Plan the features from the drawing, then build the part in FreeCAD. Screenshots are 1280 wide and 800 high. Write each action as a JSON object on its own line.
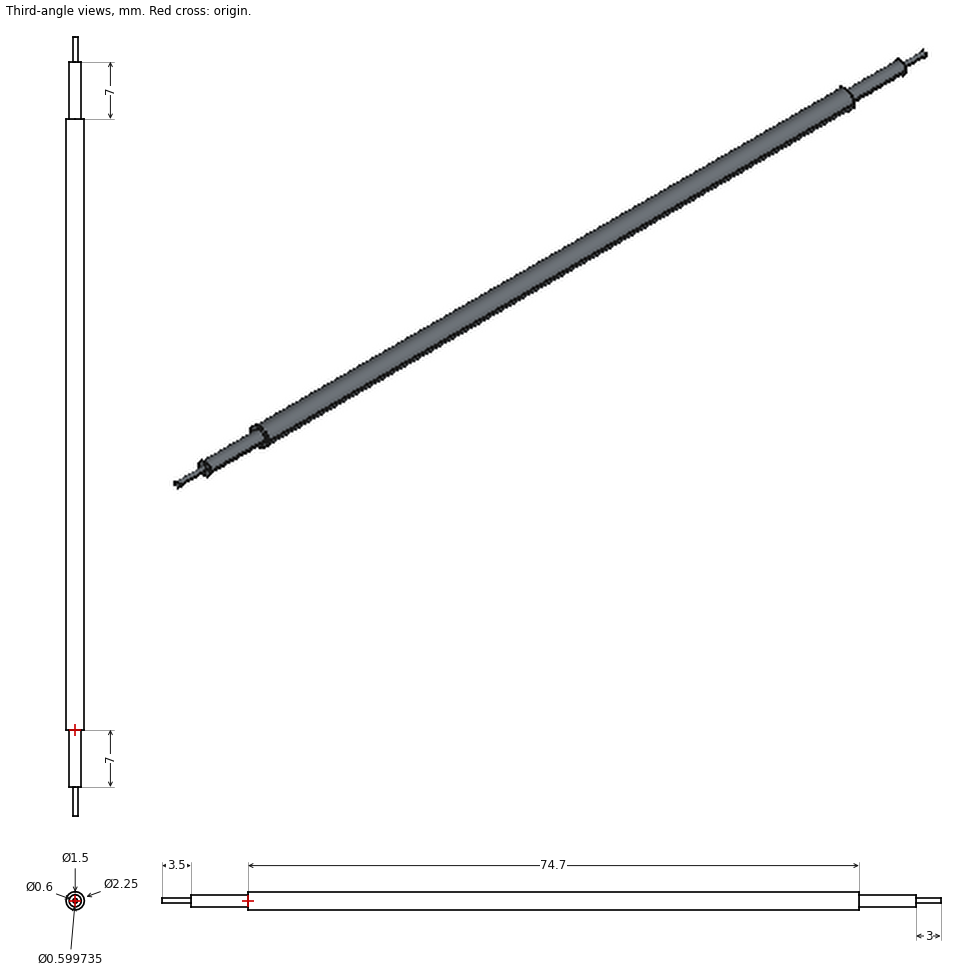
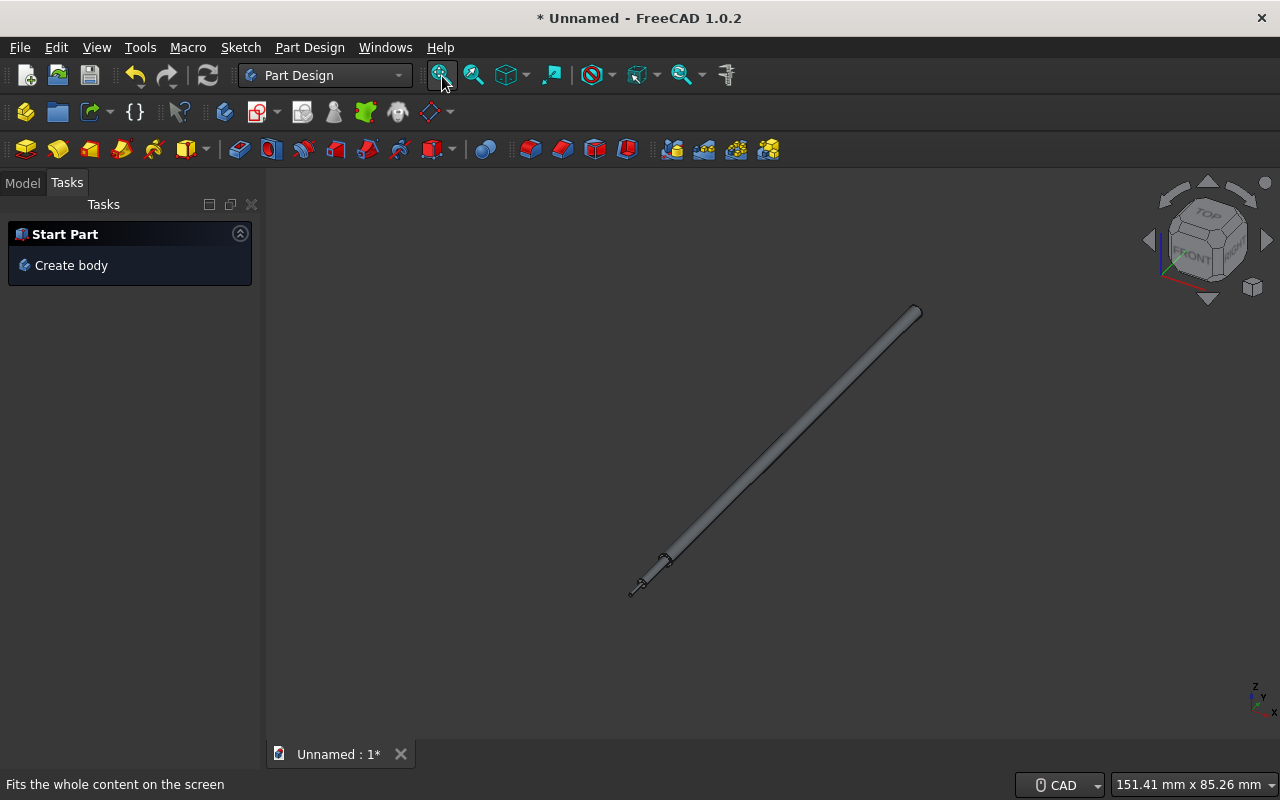
{"action": "left_click", "coordinate": [23, 182]}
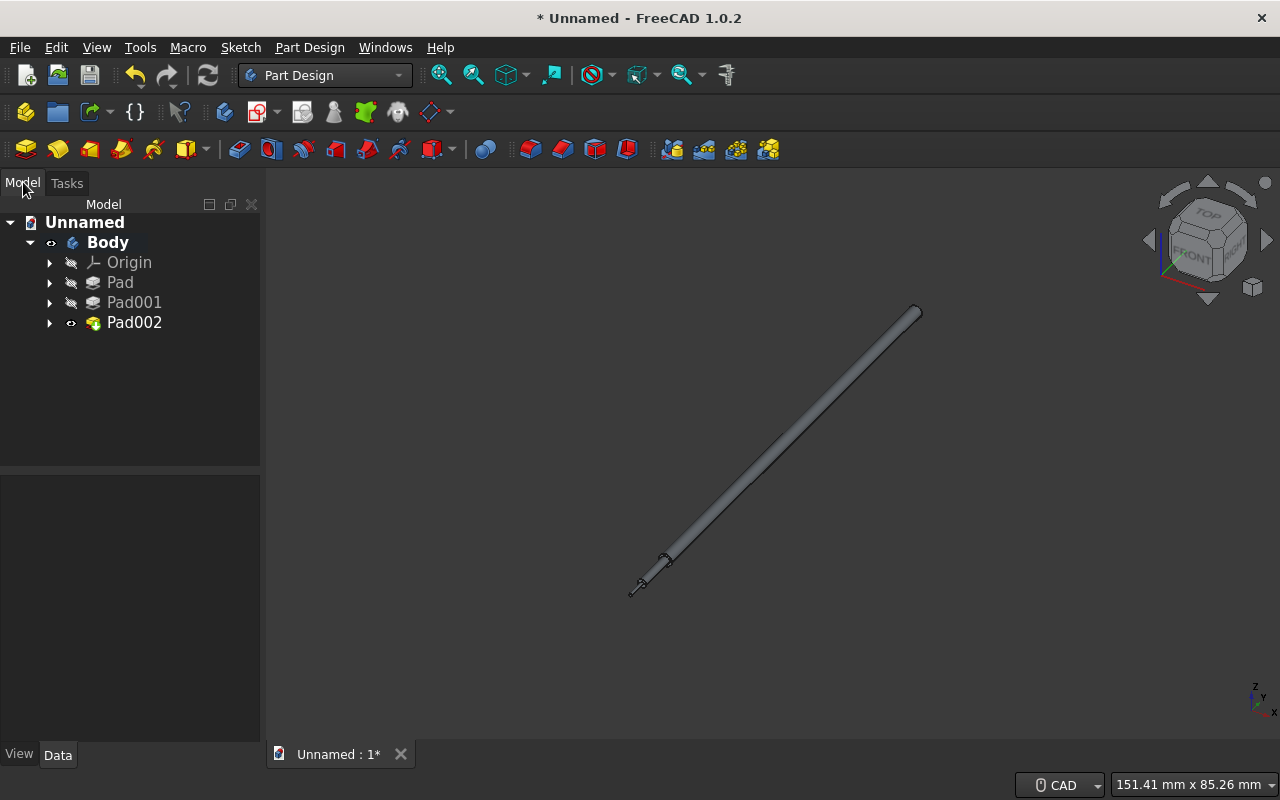
{"action": "left_click", "coordinate": [50, 263]}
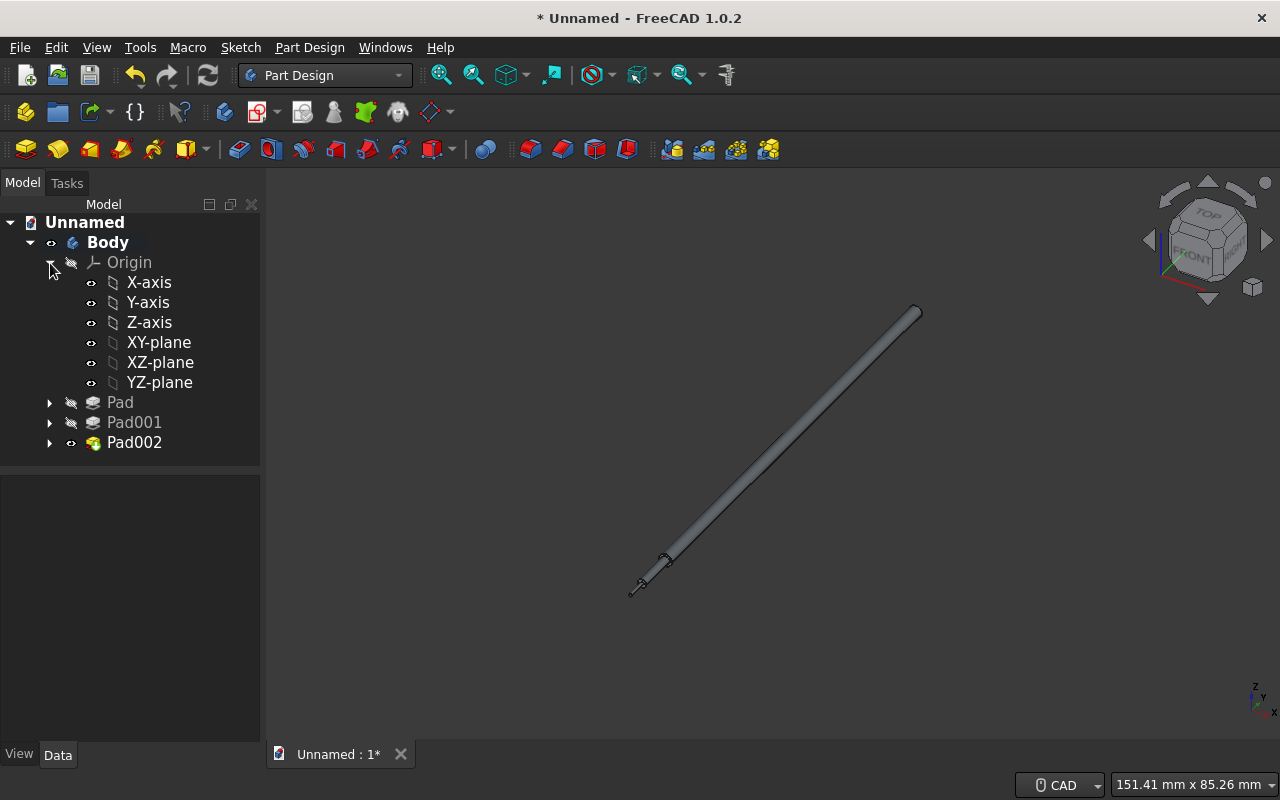
{"action": "left_click", "coordinate": [136, 363]}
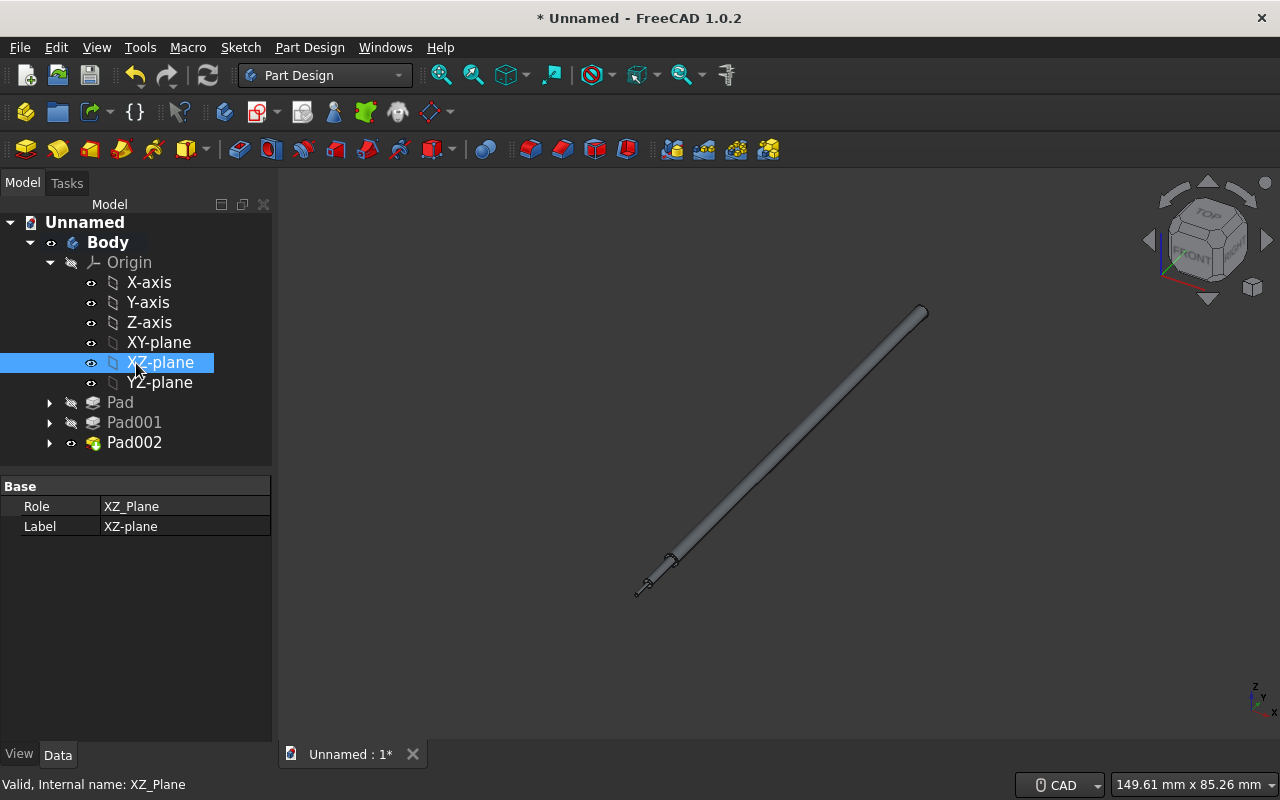
{"action": "left_click", "coordinate": [430, 112]}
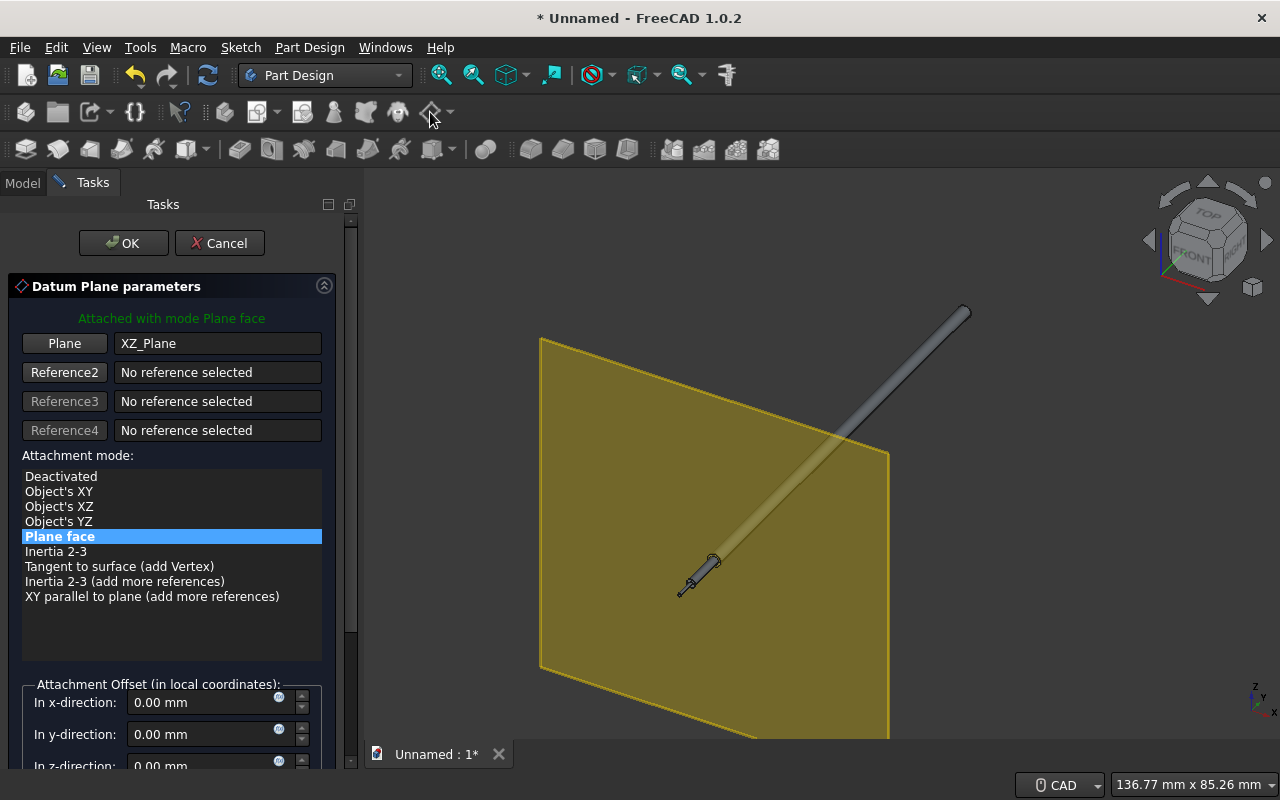
{"action": "scroll", "coordinate": [351, 491], "scroll_direction": "down", "scroll_amount": 2}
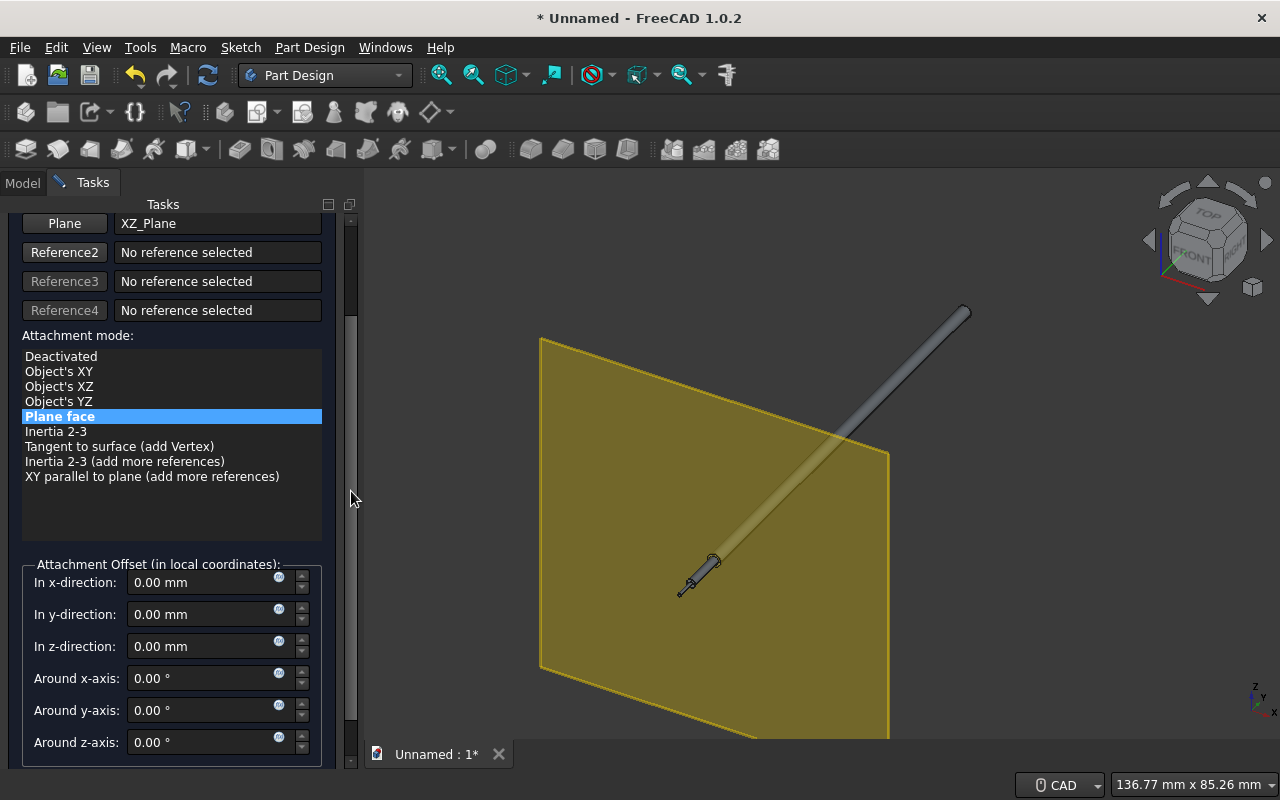
{"action": "triple_click", "coordinate": [210, 646]}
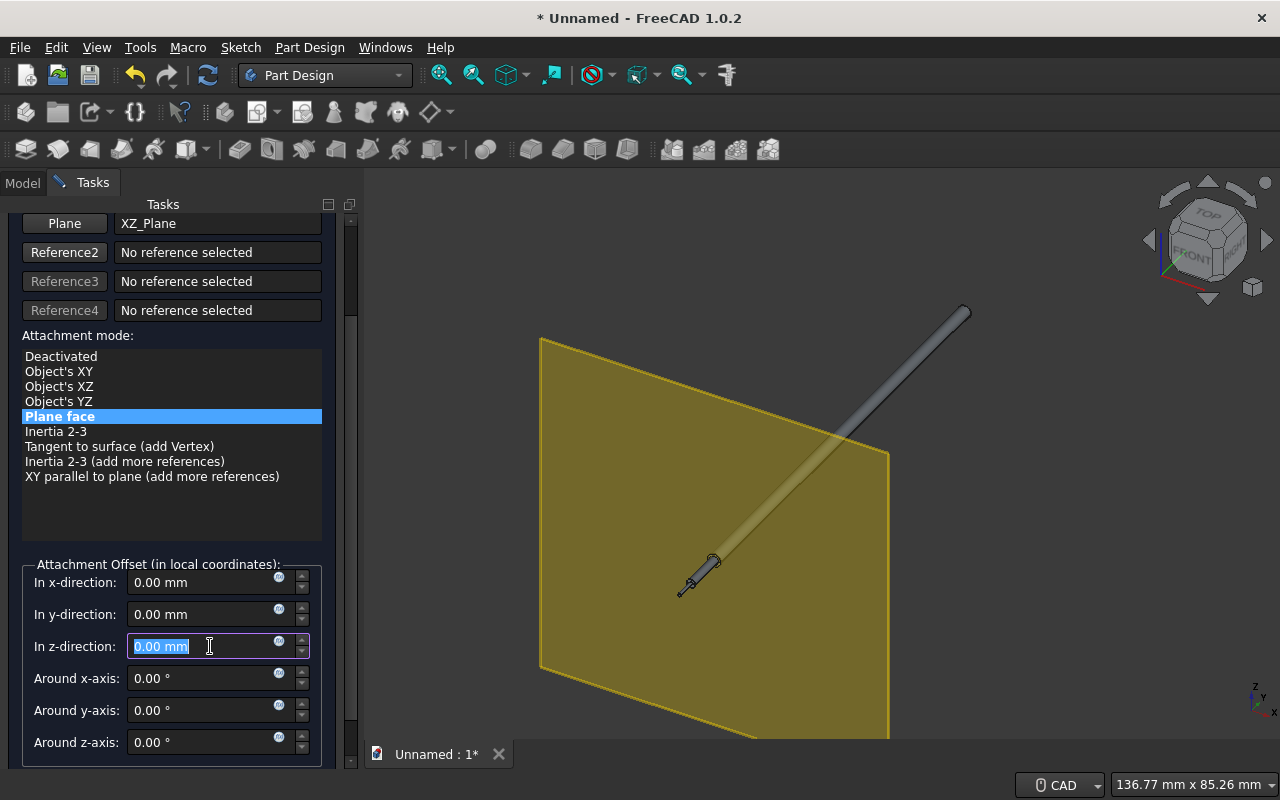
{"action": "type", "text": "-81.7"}
{"action": "key", "text": "Tab"}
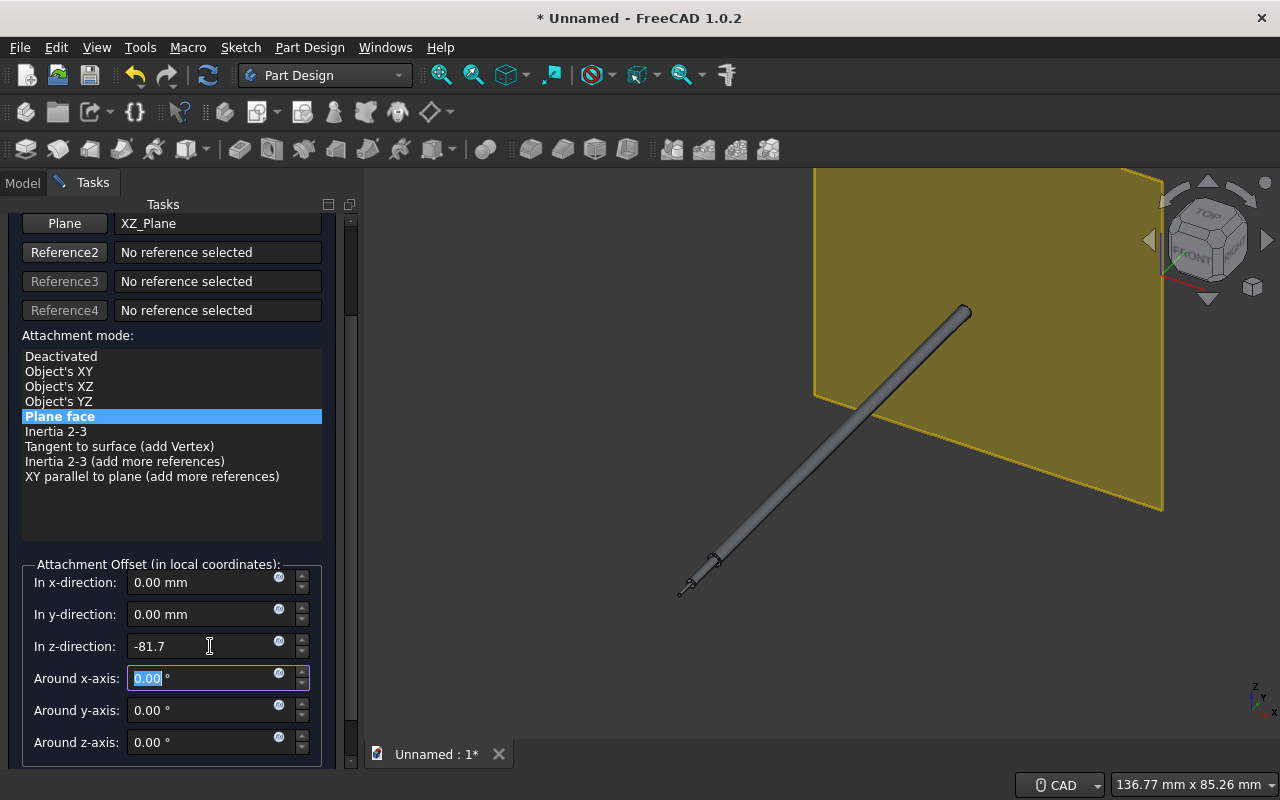
{"action": "scroll", "coordinate": [351, 491], "scroll_direction": "up", "scroll_amount": 3}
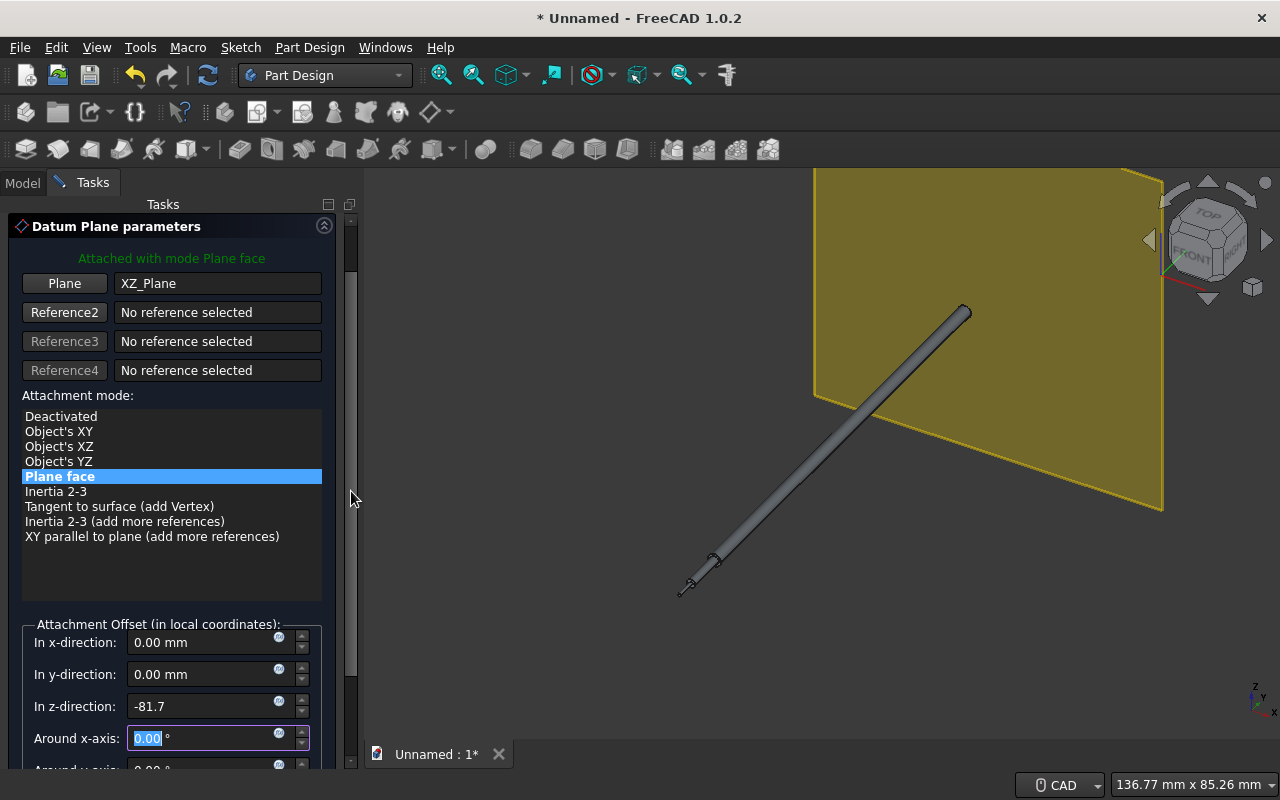
{"action": "left_click", "coordinate": [124, 243]}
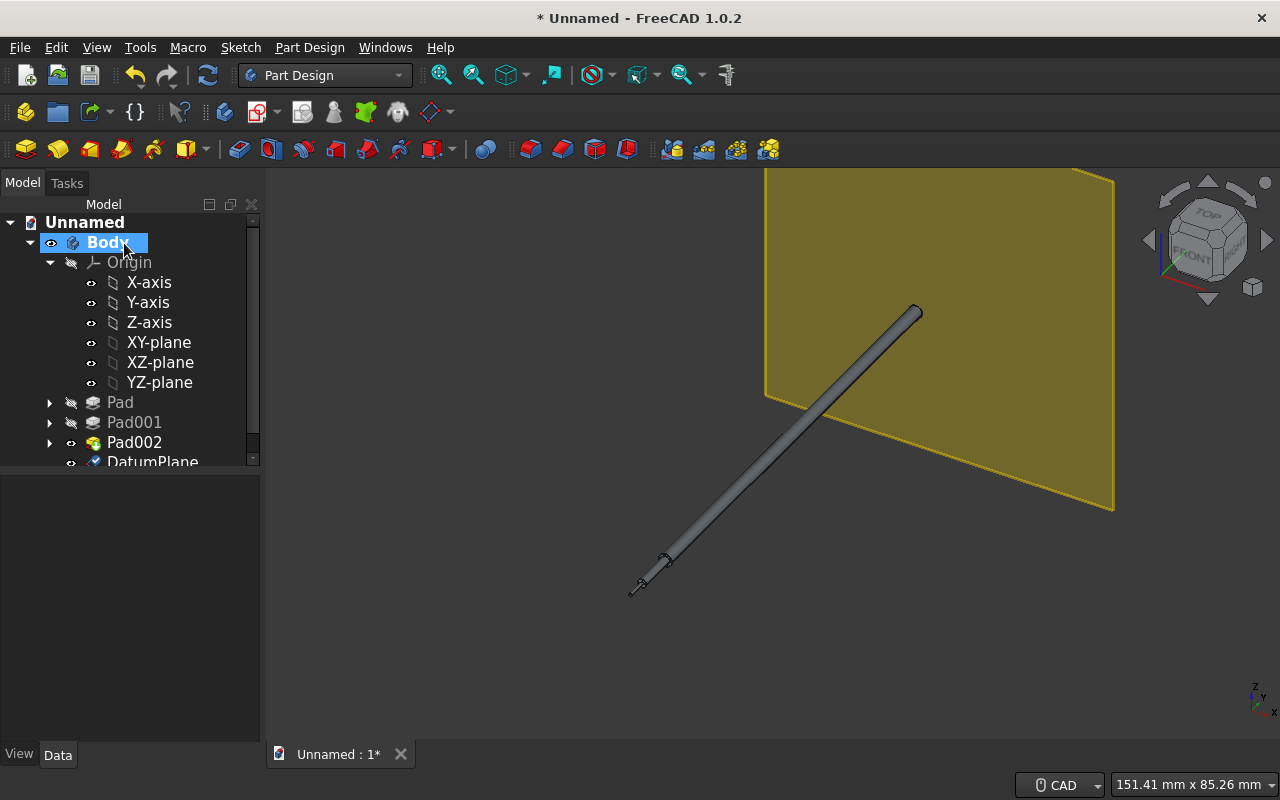
{"action": "left_click", "coordinate": [116, 463]}